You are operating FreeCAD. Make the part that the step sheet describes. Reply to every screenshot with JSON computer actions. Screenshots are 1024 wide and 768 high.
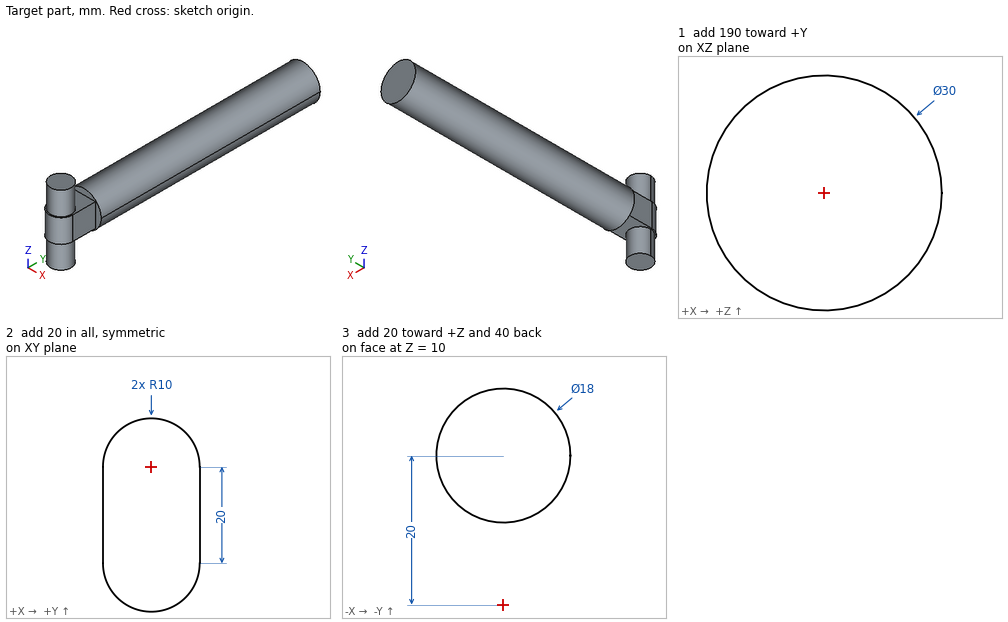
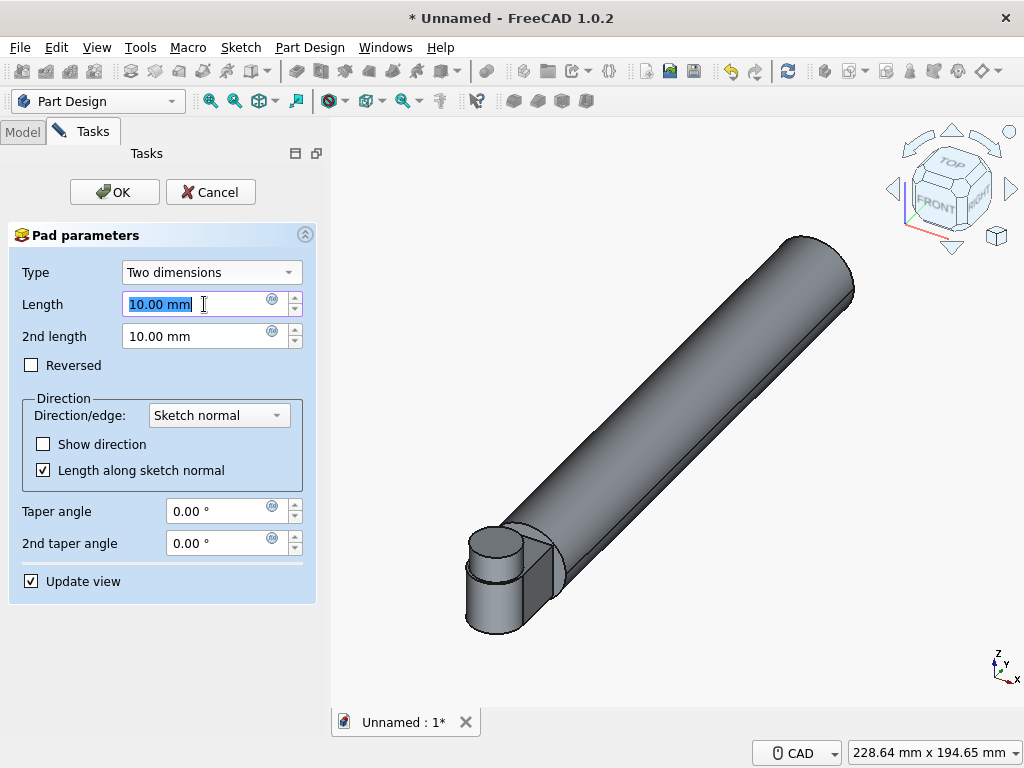
{"action": "type", "text": "20"}
{"action": "key", "text": "Tab"}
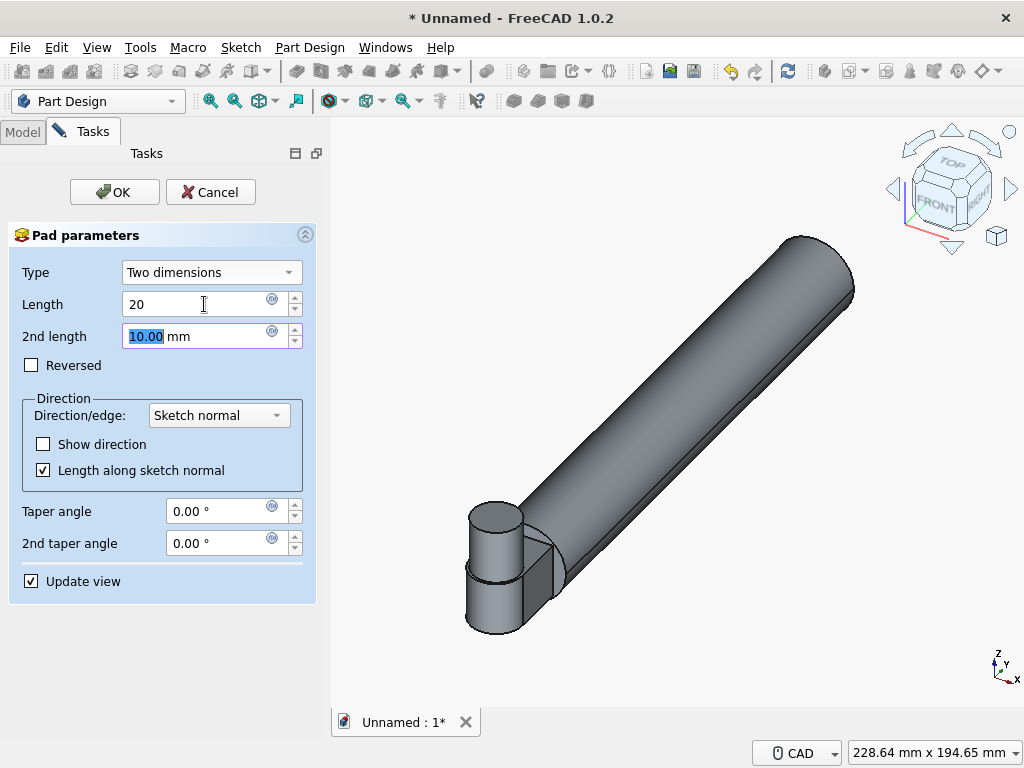
{"action": "type", "text": "40"}
{"action": "key", "text": "Tab"}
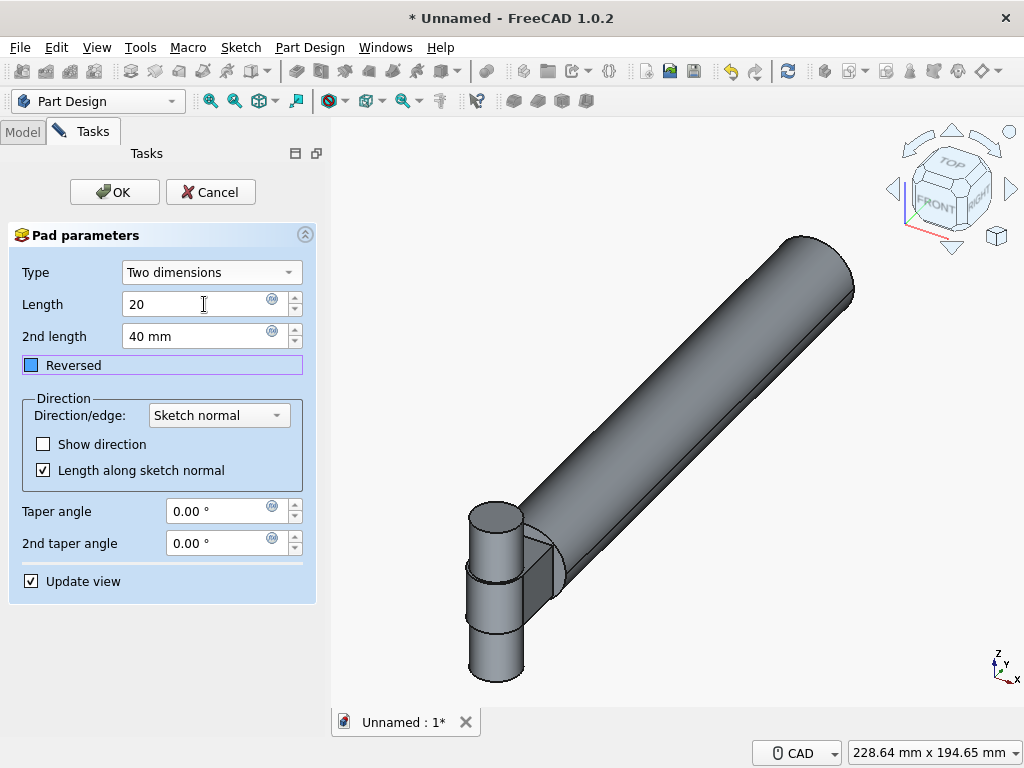
{"action": "left_click", "coordinate": [115, 192]}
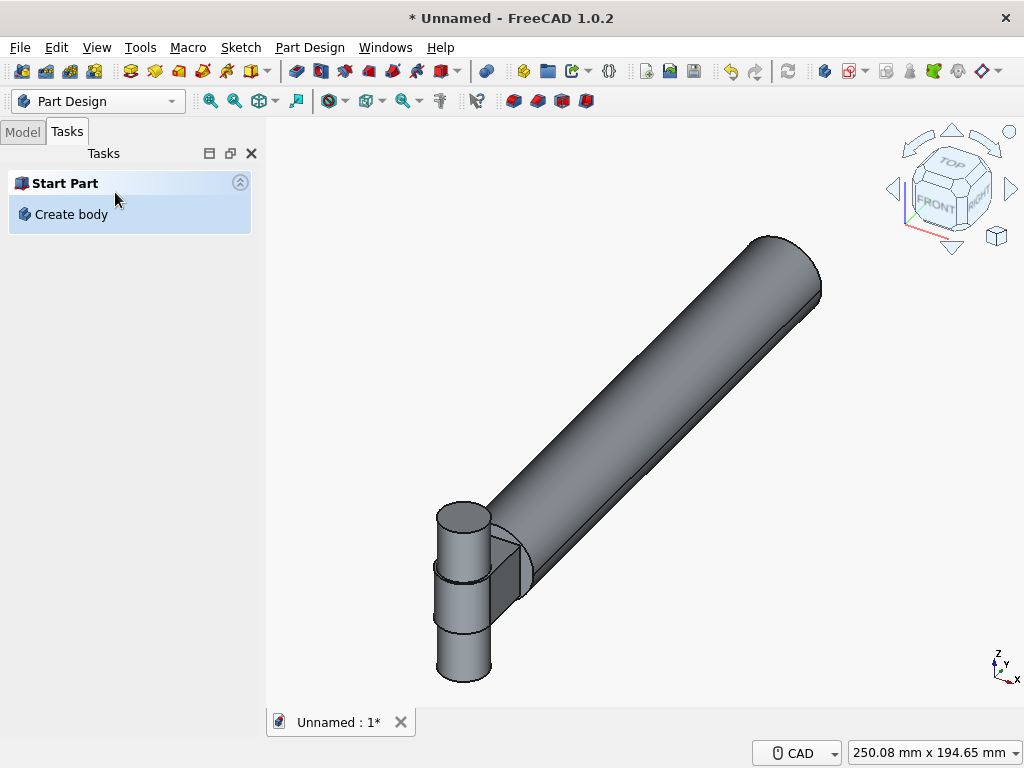
{"action": "key", "text": "0"}